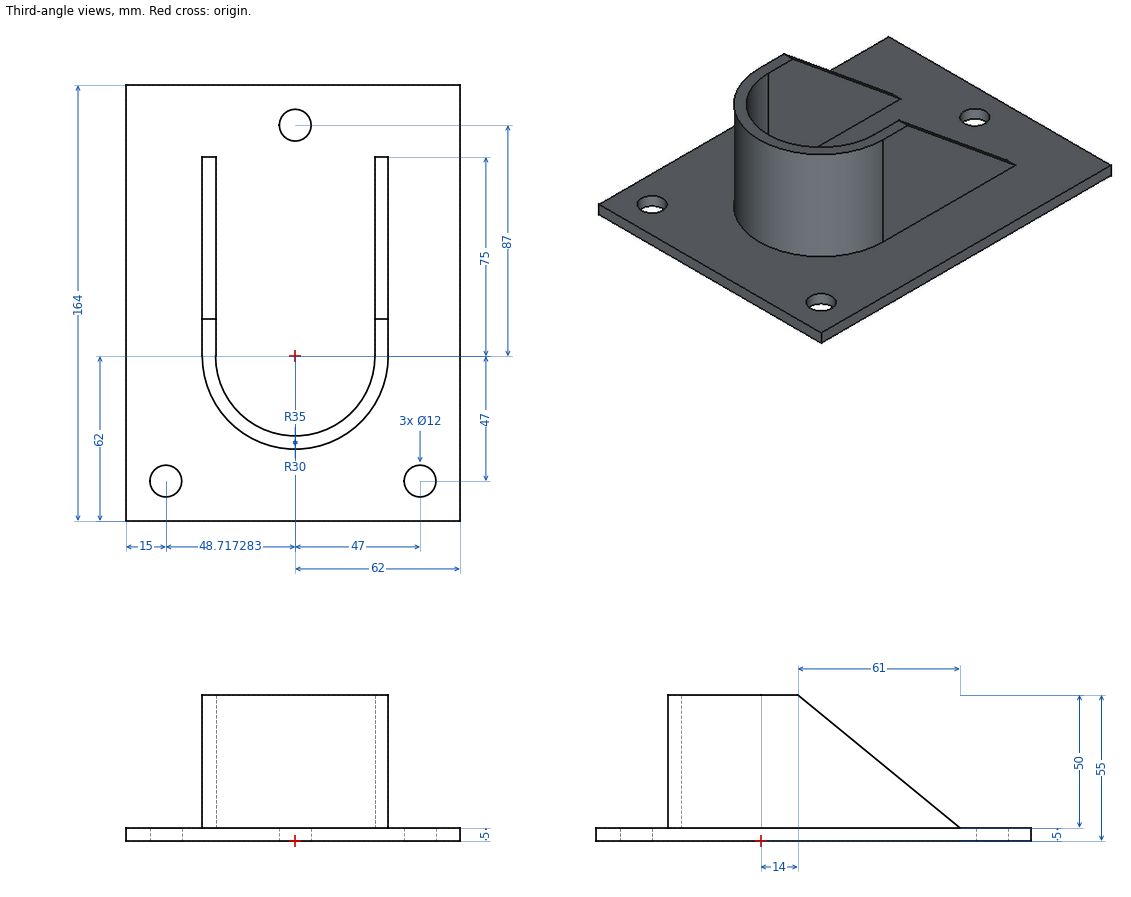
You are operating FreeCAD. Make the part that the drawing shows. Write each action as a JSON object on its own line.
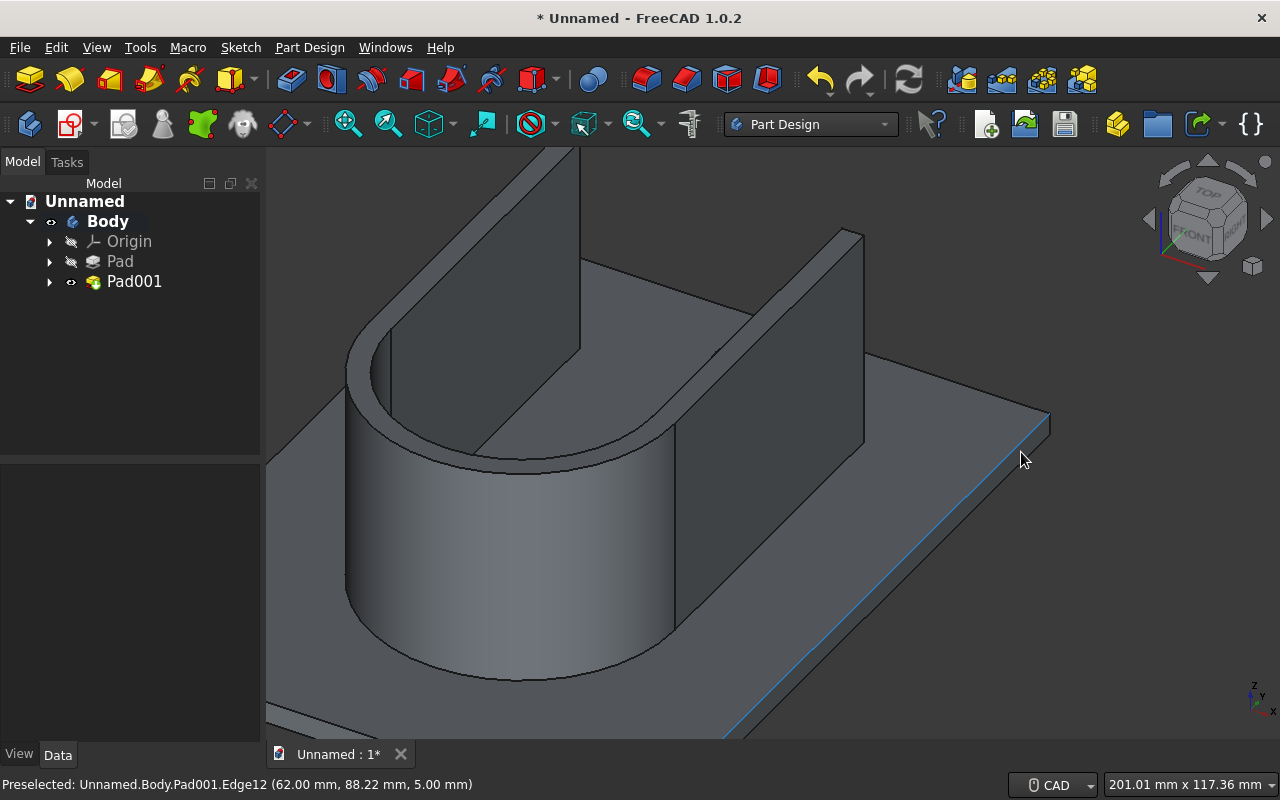
{"action": "left_click", "coordinate": [350, 124]}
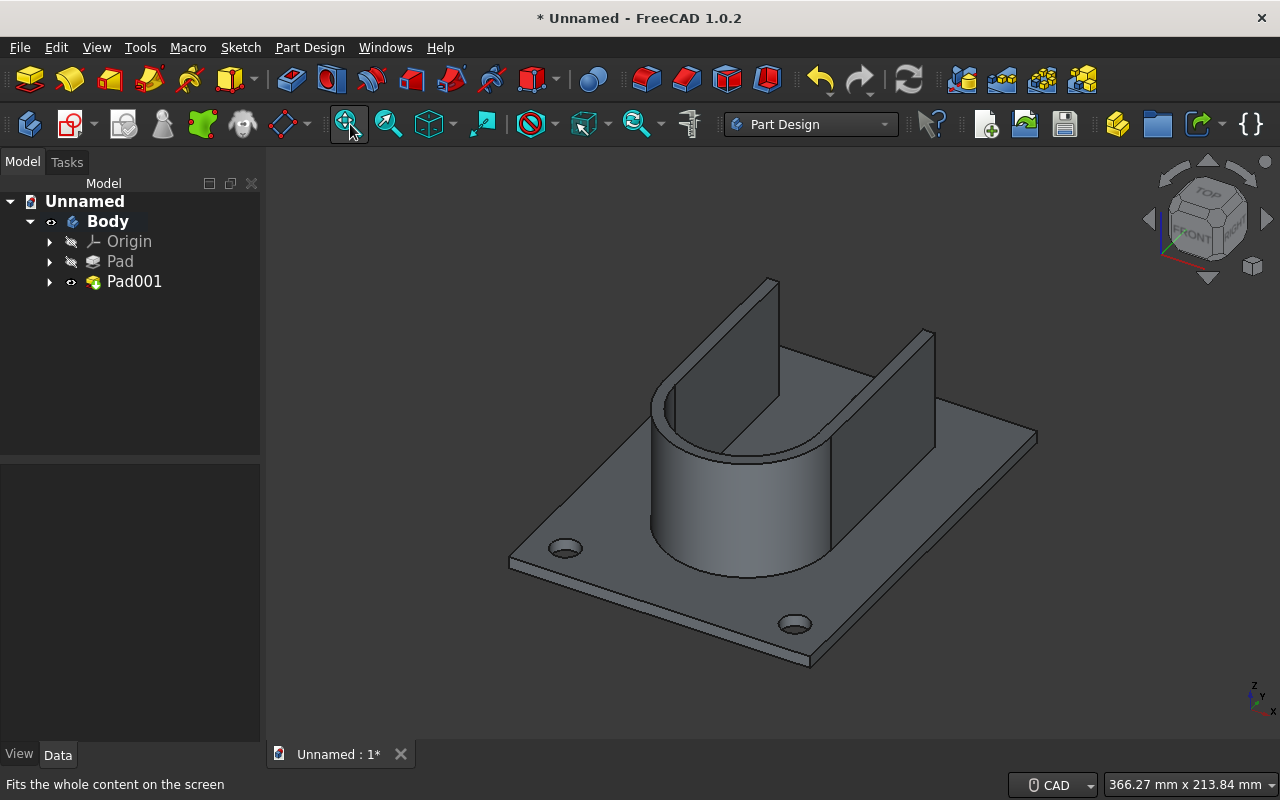
{"action": "key", "text": "0"}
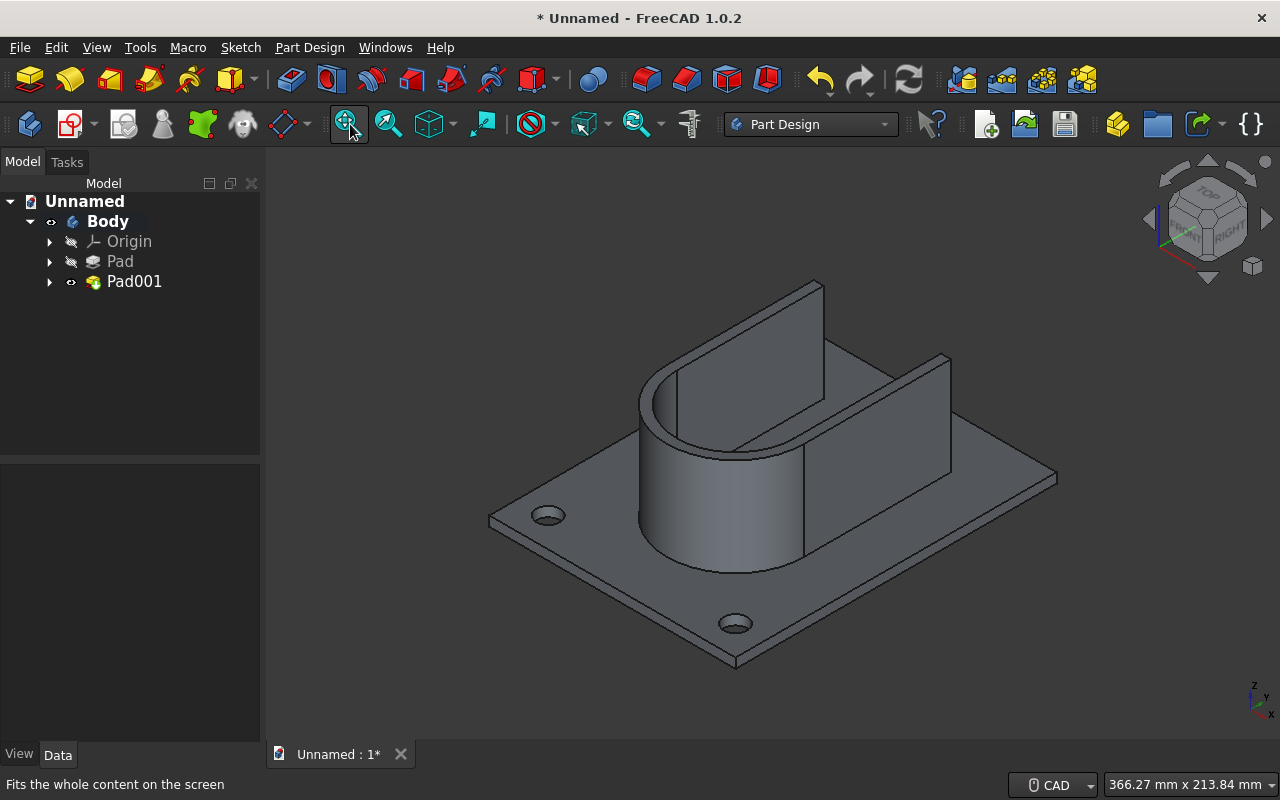
{"action": "scroll", "coordinate": [1034, 490], "scroll_direction": "up", "scroll_amount": 3}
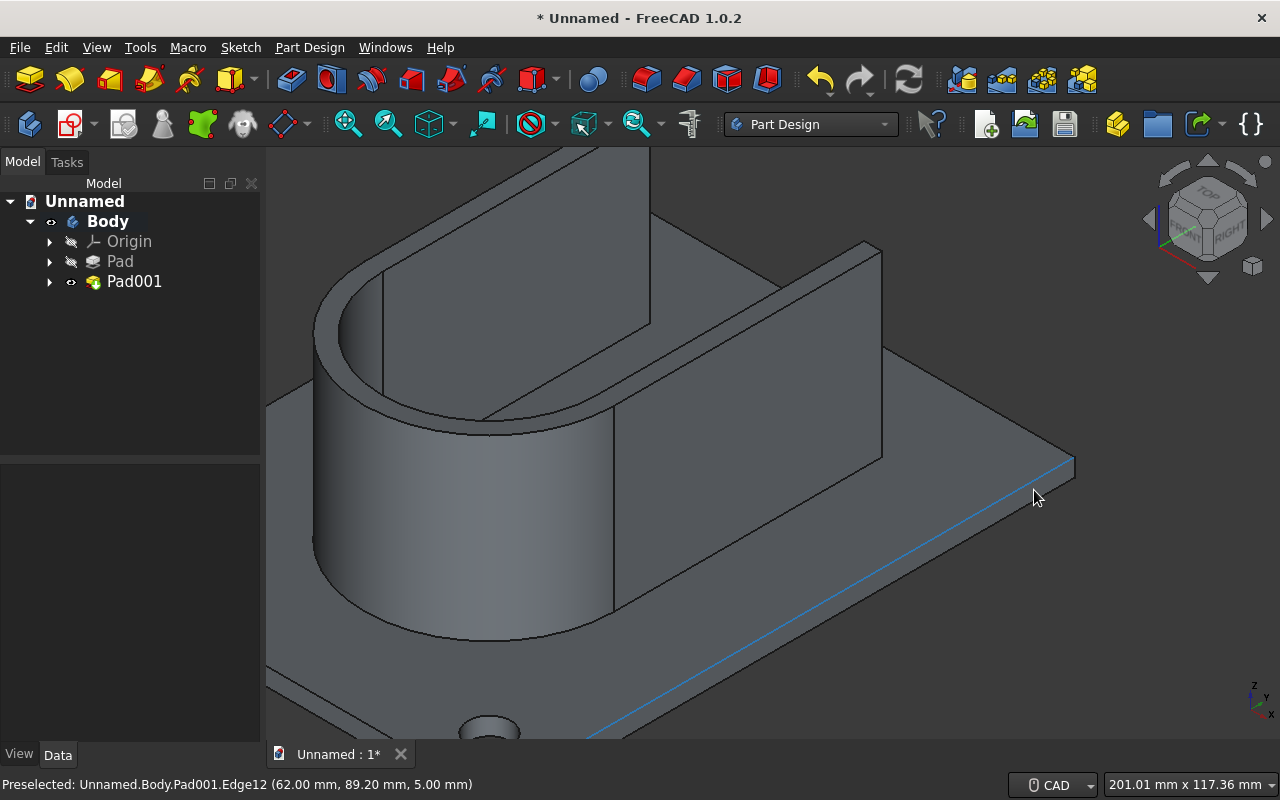
{"action": "left_click", "coordinate": [1033, 491]}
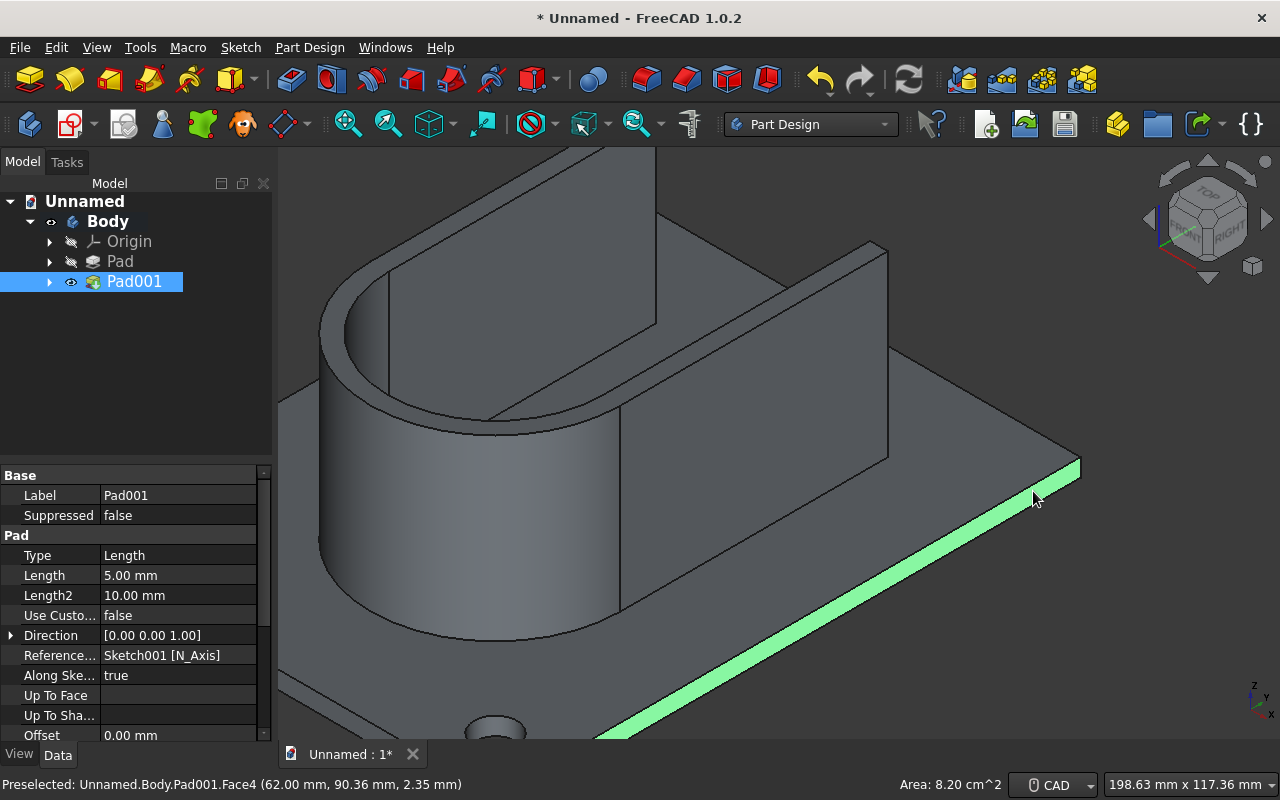
{"action": "left_click", "coordinate": [70, 124]}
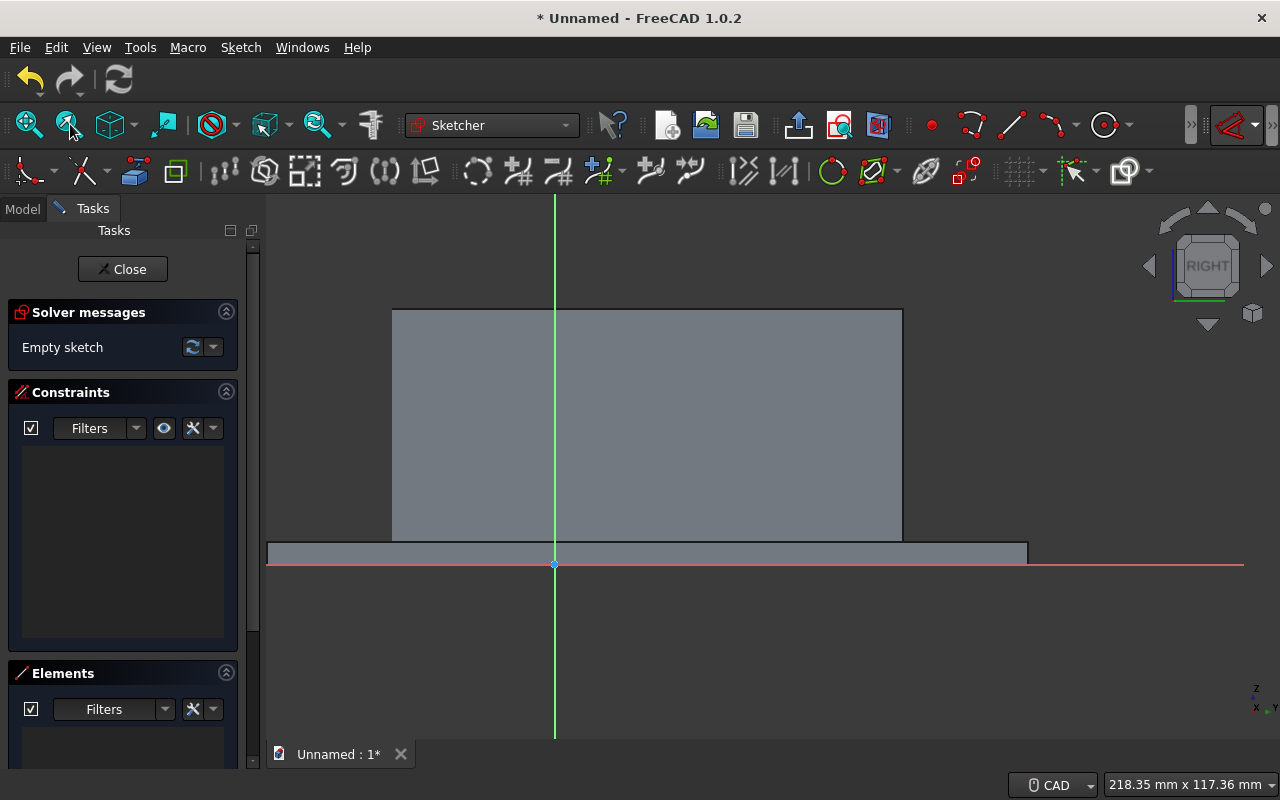
{"action": "scroll", "coordinate": [778, 377], "scroll_direction": "up", "scroll_amount": 2}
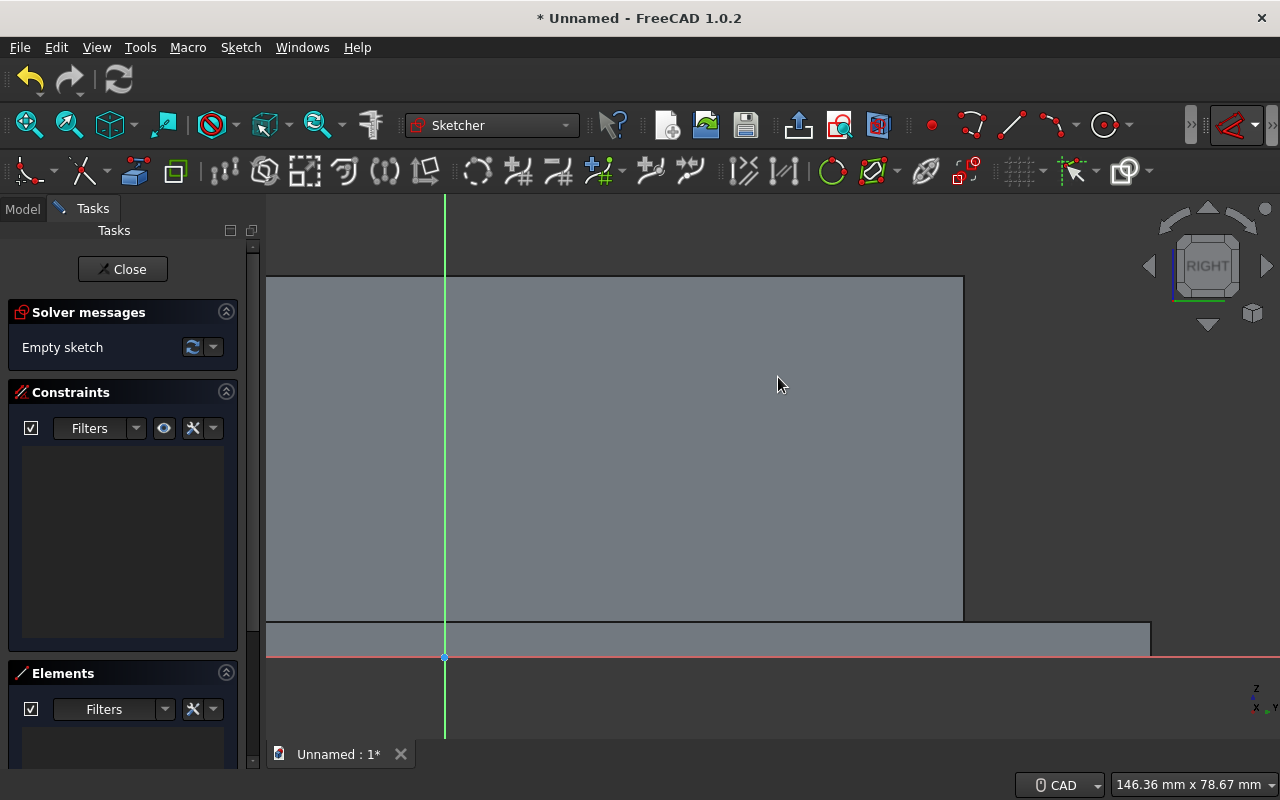
{"action": "left_click", "coordinate": [972, 126]}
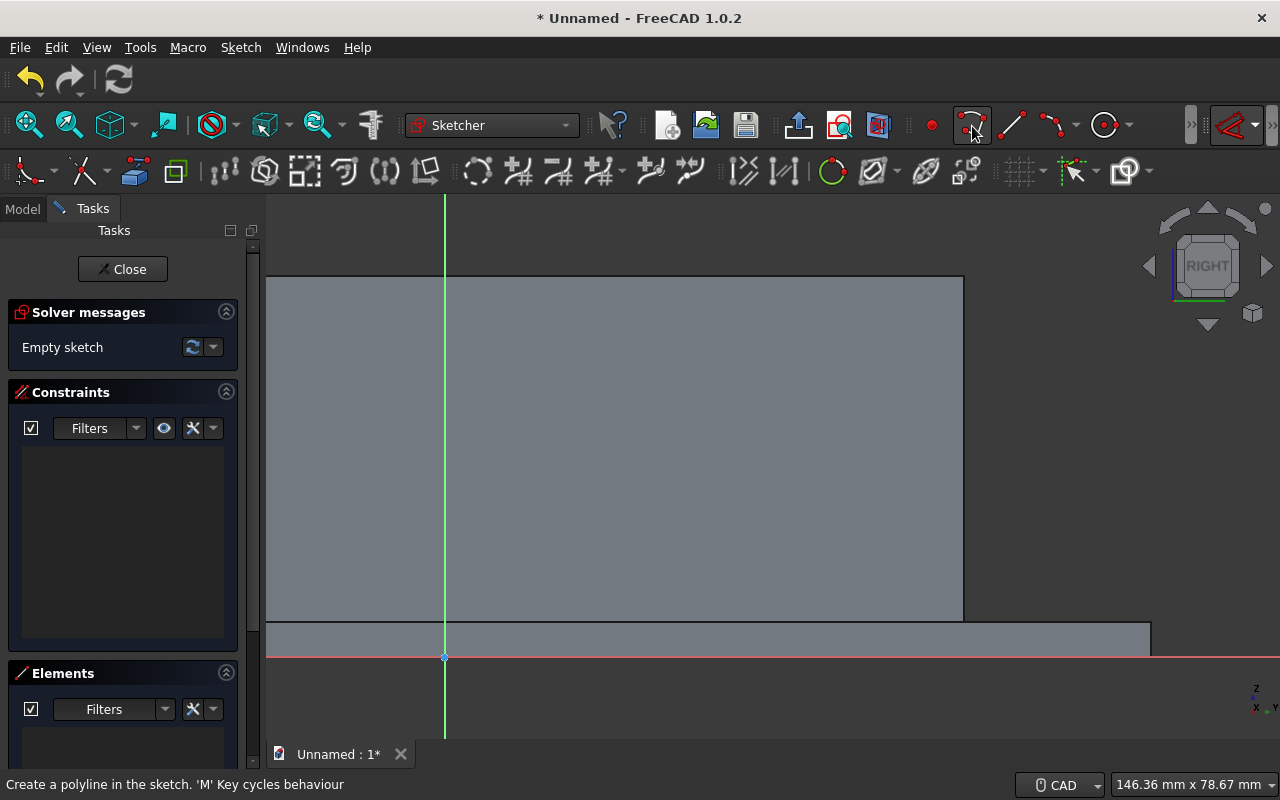
{"action": "left_click", "coordinate": [542, 276]}
{"action": "left_click", "coordinate": [964, 622]}
{"action": "left_click", "coordinate": [964, 276]}
{"action": "left_click", "coordinate": [542, 277]}
{"action": "key", "text": "Escape"}
{"action": "key", "text": "Escape"}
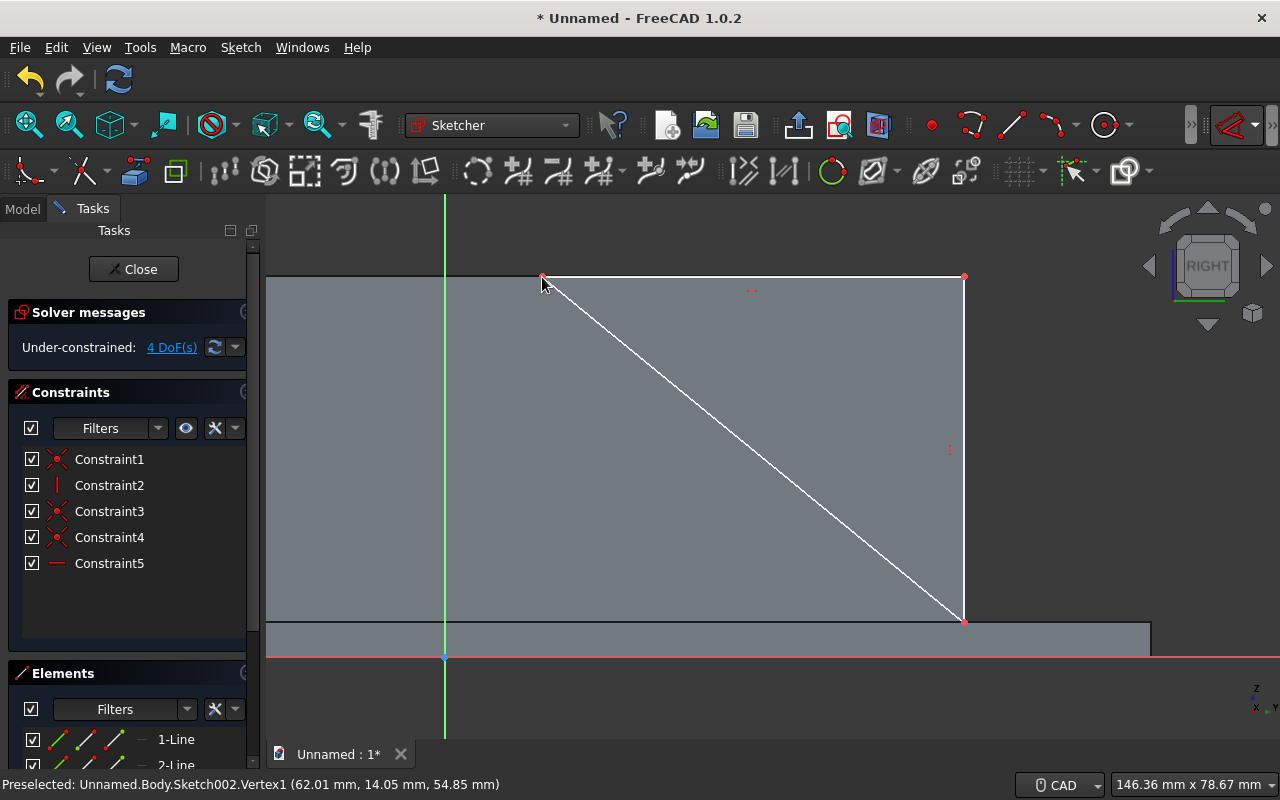
{"action": "left_click", "coordinate": [964, 519]}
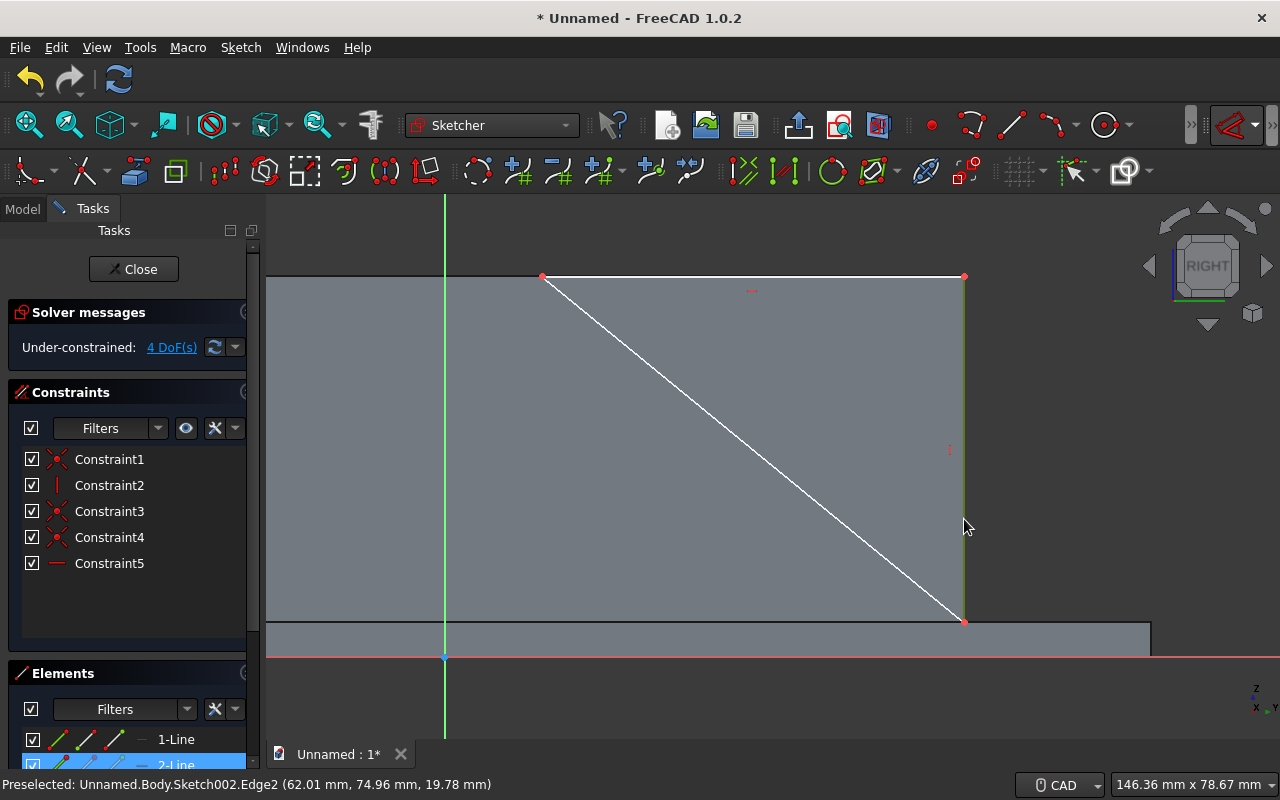
{"action": "key", "text": "i"}